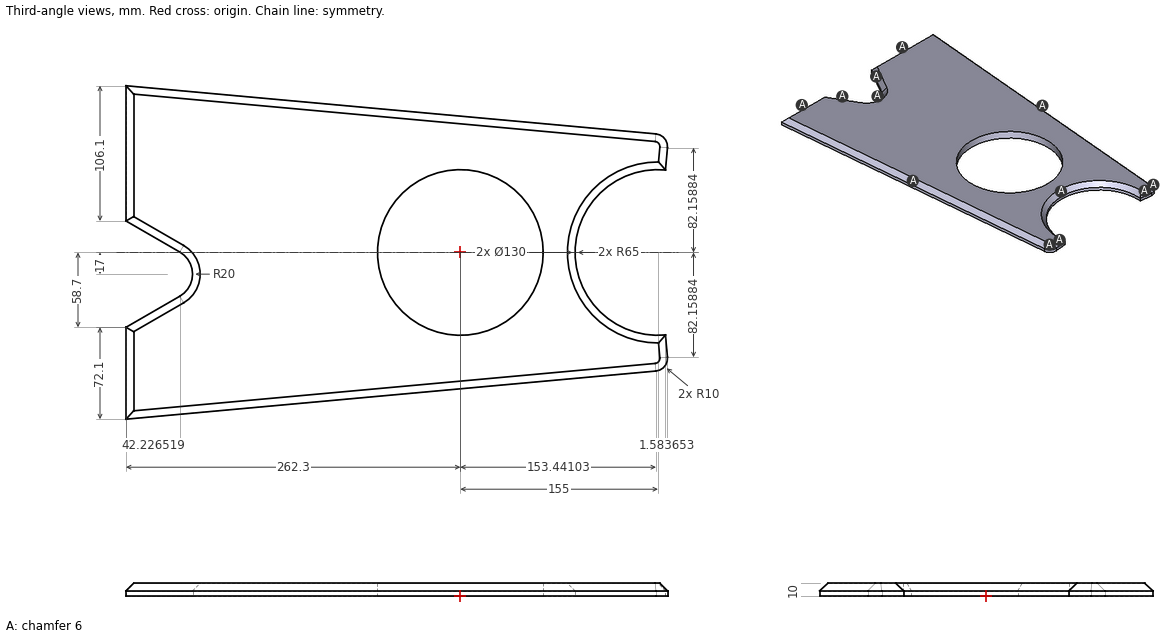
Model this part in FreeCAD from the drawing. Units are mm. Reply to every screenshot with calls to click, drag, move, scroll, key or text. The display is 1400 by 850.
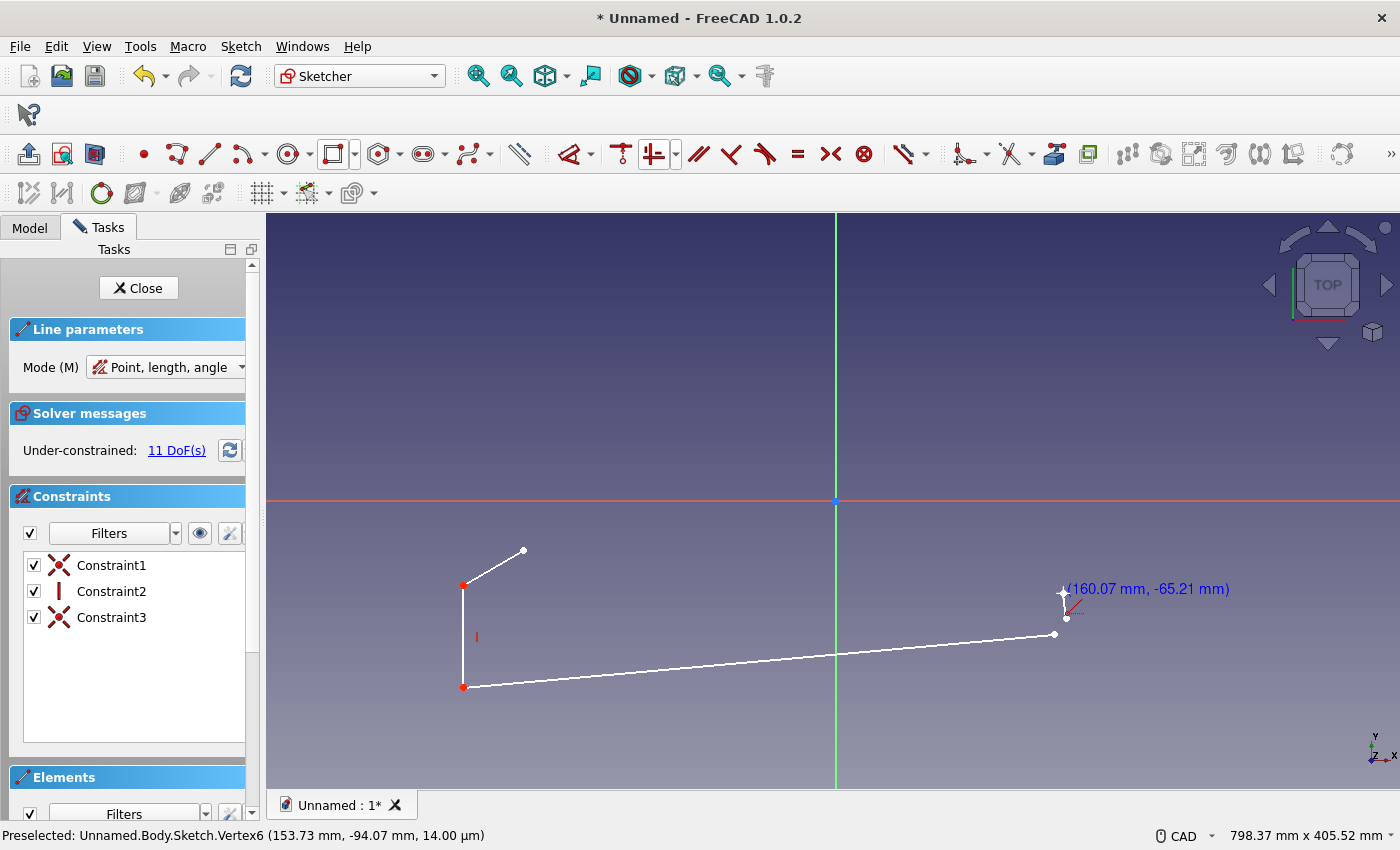
click(1064, 409)
click(1067, 385)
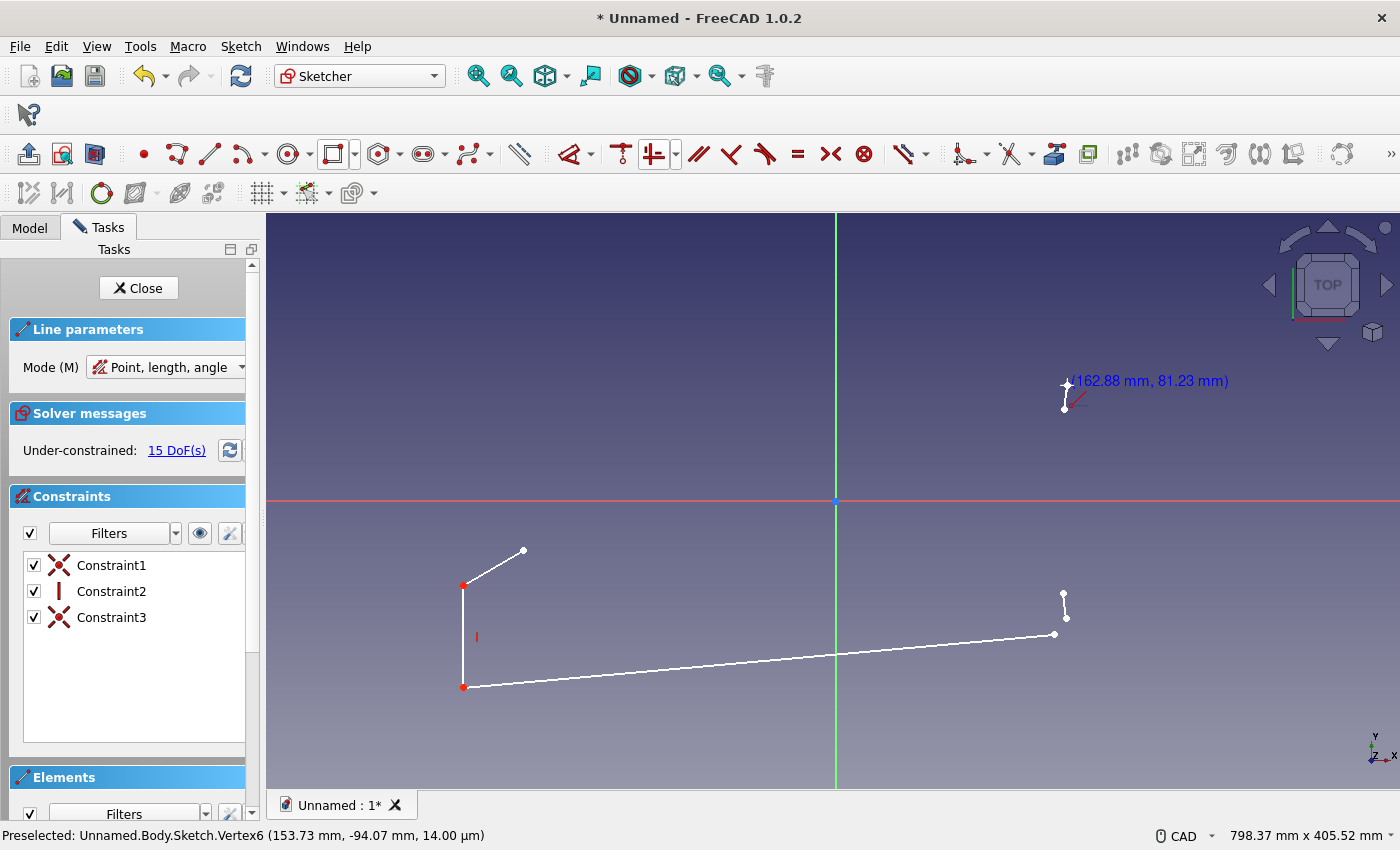
click(177, 154)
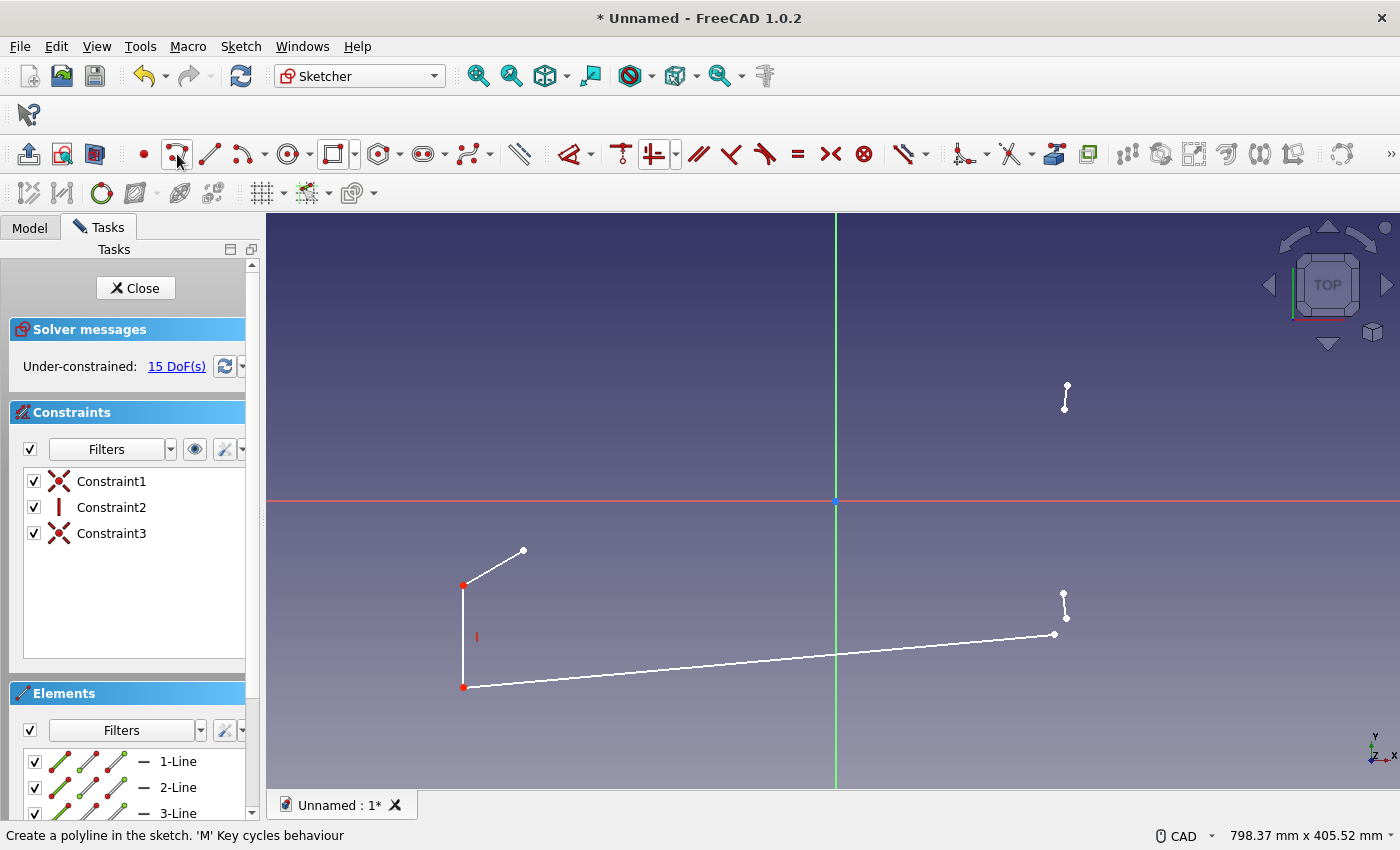
click(1054, 369)
click(463, 316)
click(463, 466)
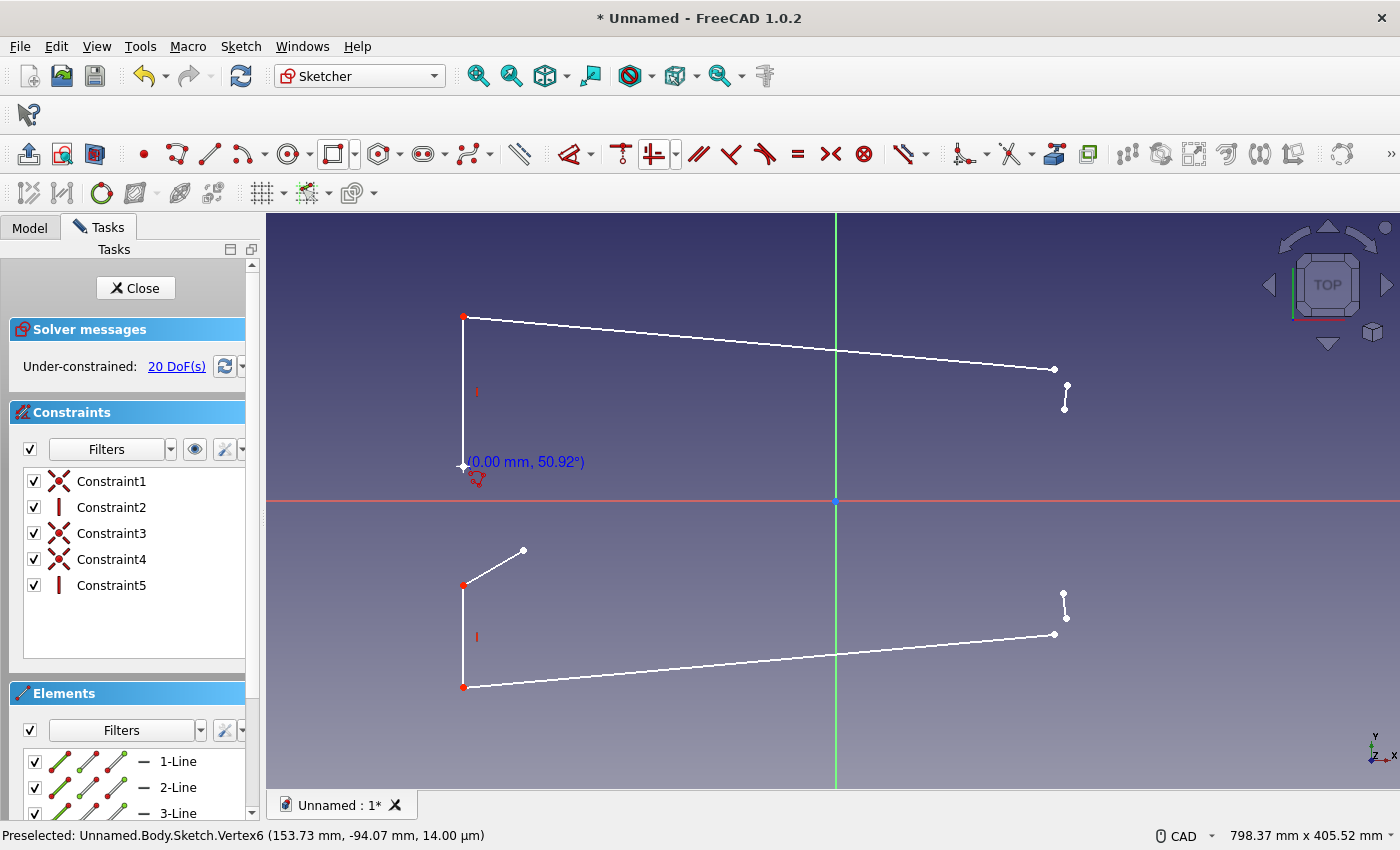
scroll(523, 501, up, 18)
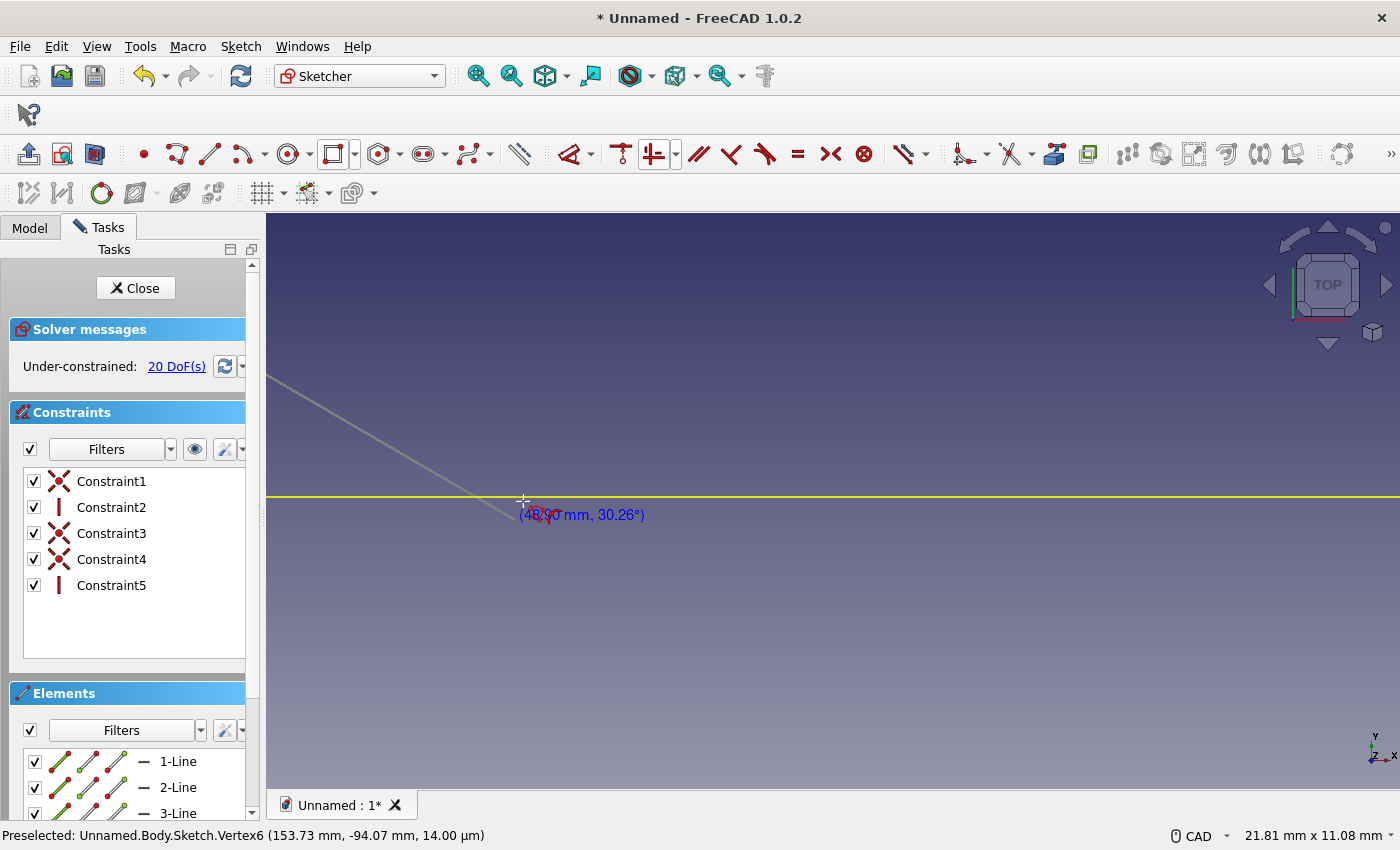
click(517, 480)
right_click(517, 480)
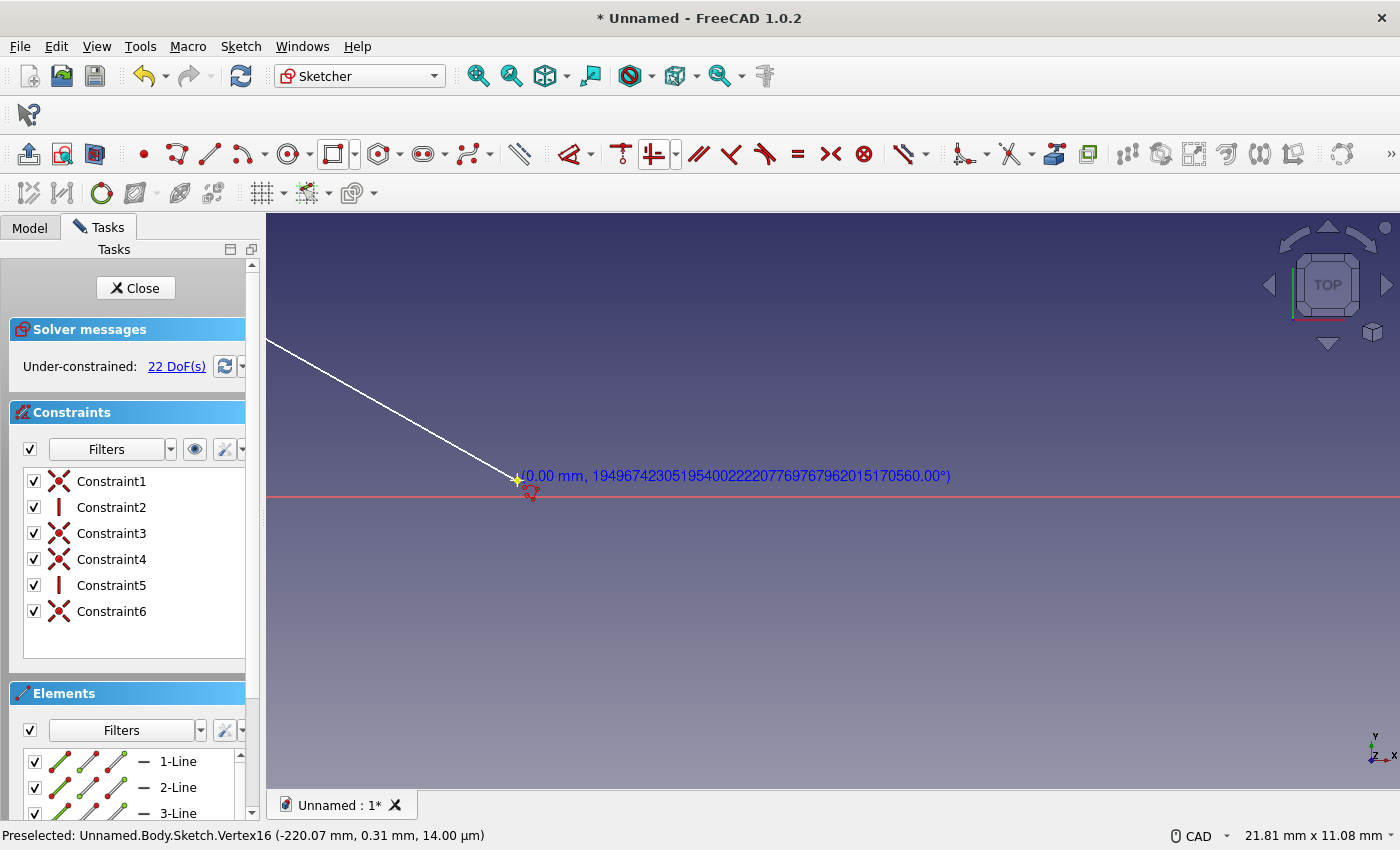
key(g)
key(3)
key(a)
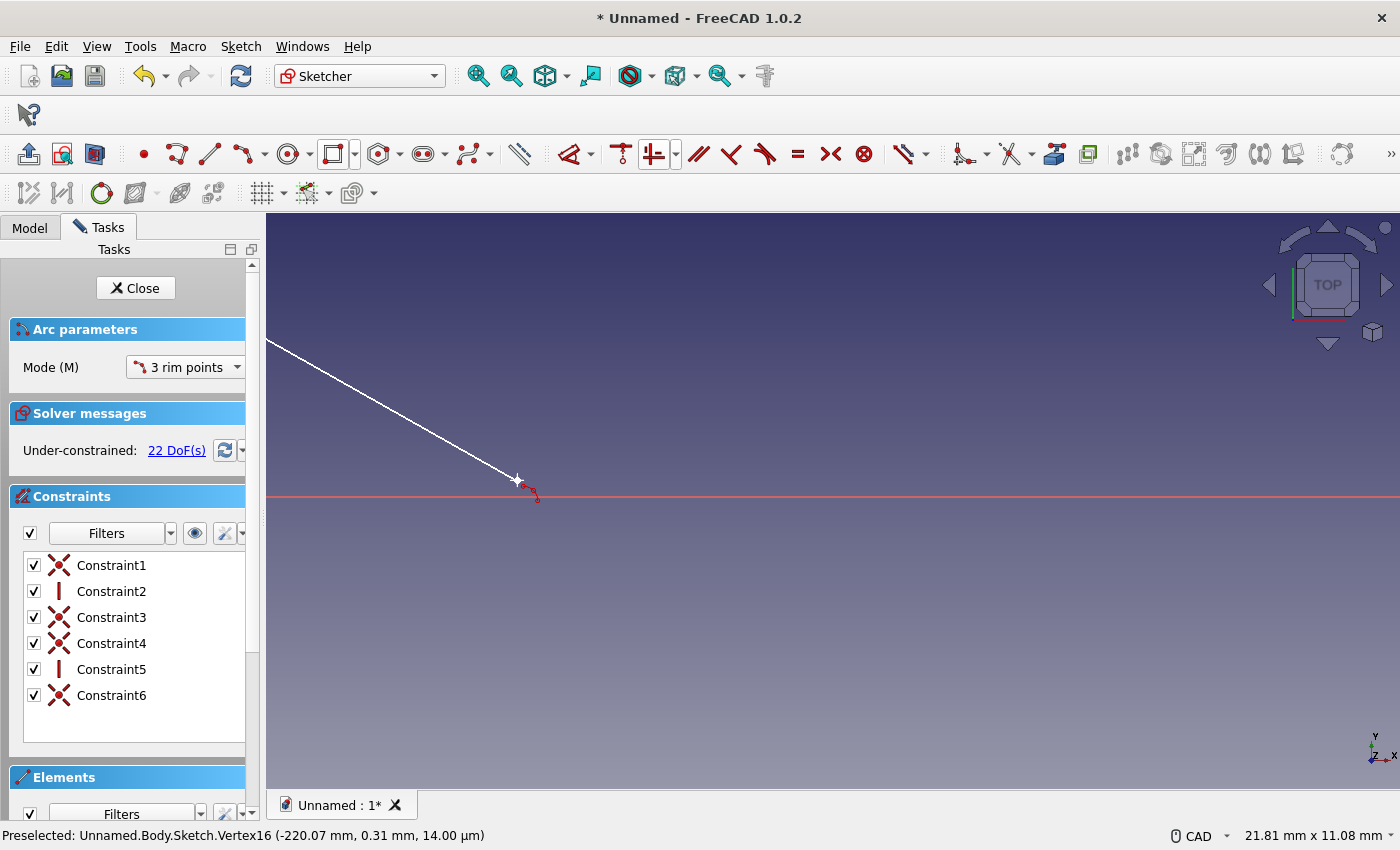
scroll(468, 501, down, 17)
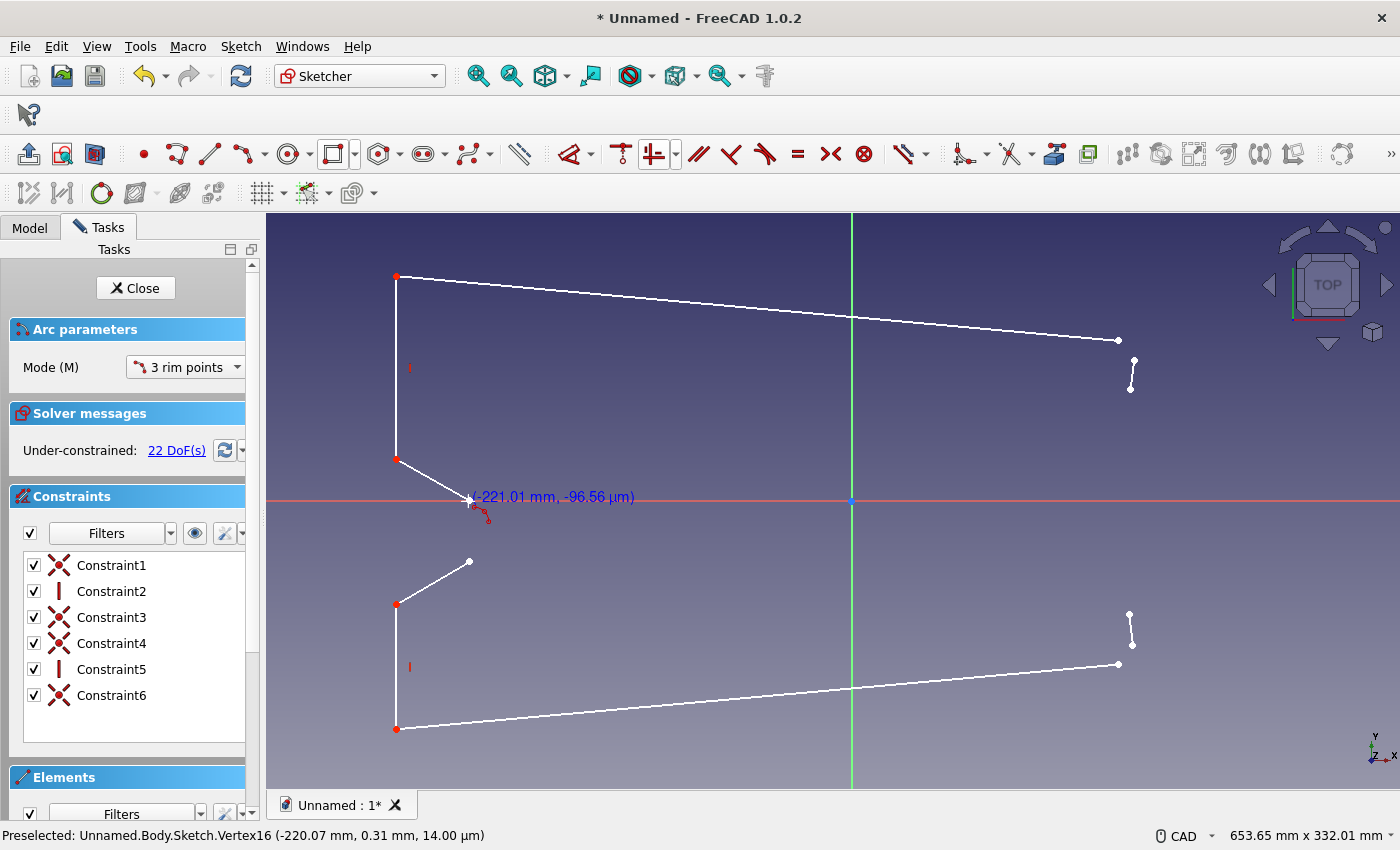
click(1118, 665)
click(1133, 645)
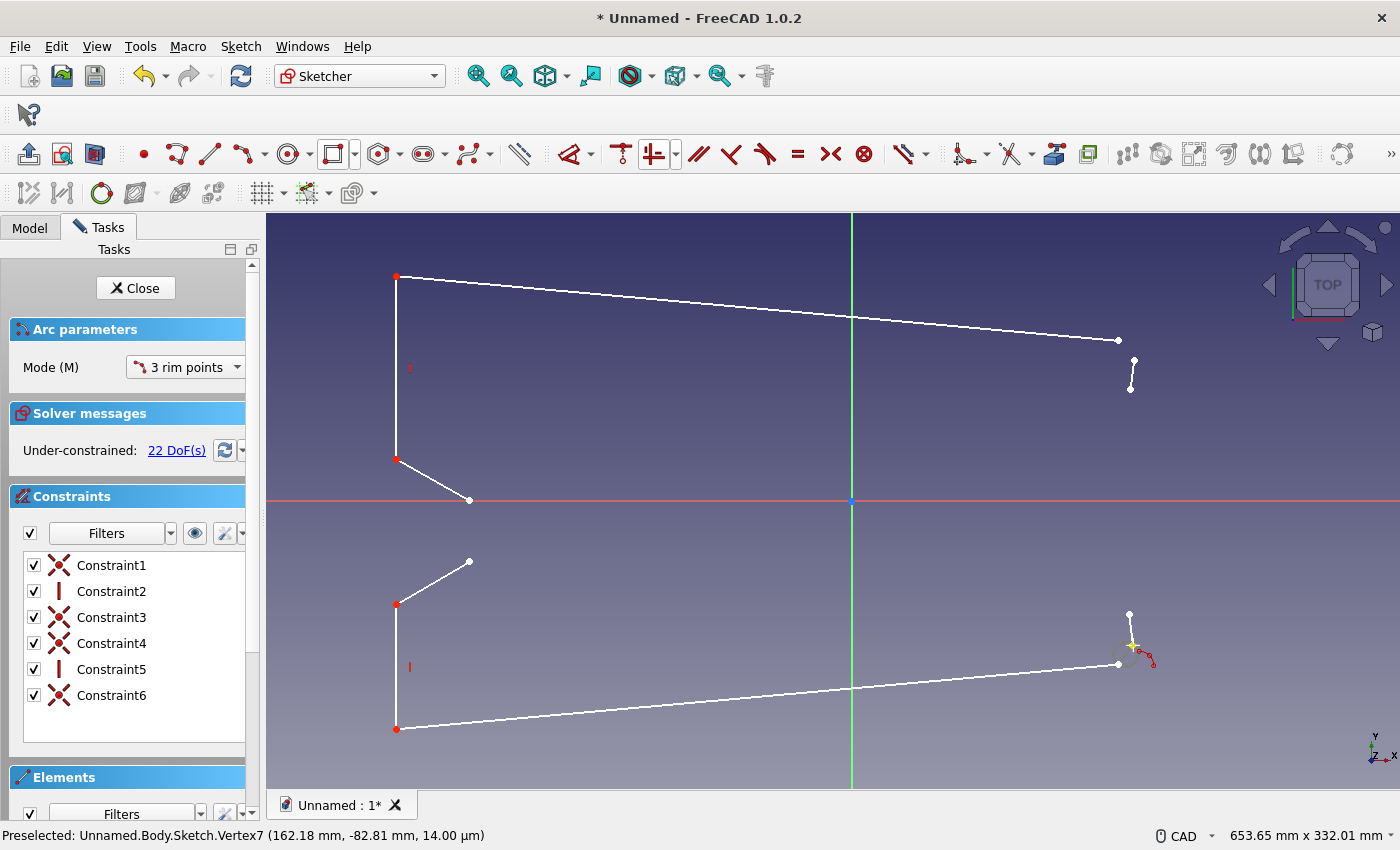
scroll(1130, 657, up, 6)